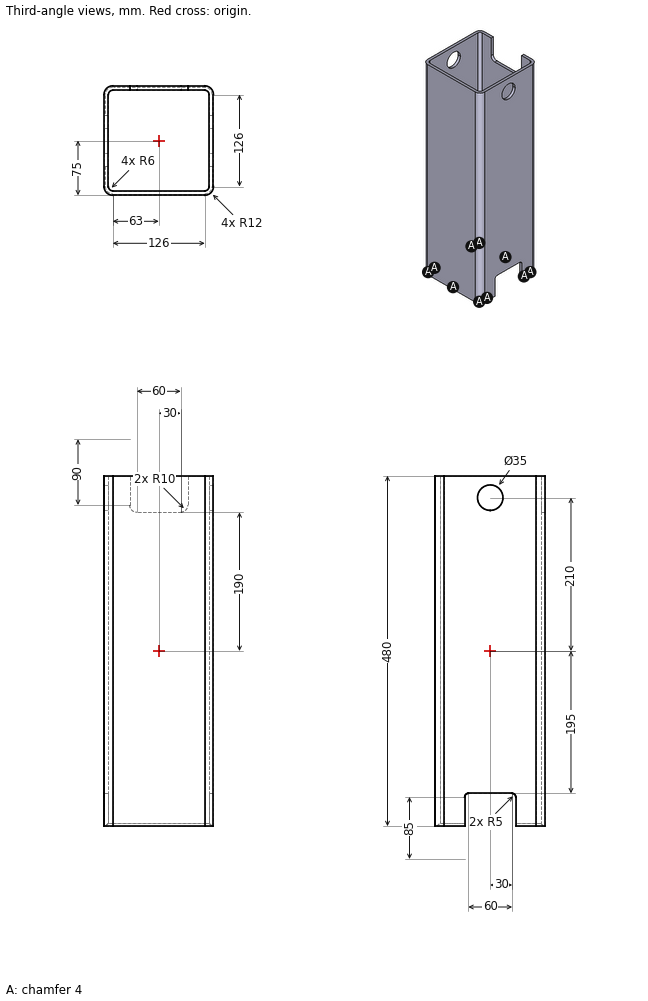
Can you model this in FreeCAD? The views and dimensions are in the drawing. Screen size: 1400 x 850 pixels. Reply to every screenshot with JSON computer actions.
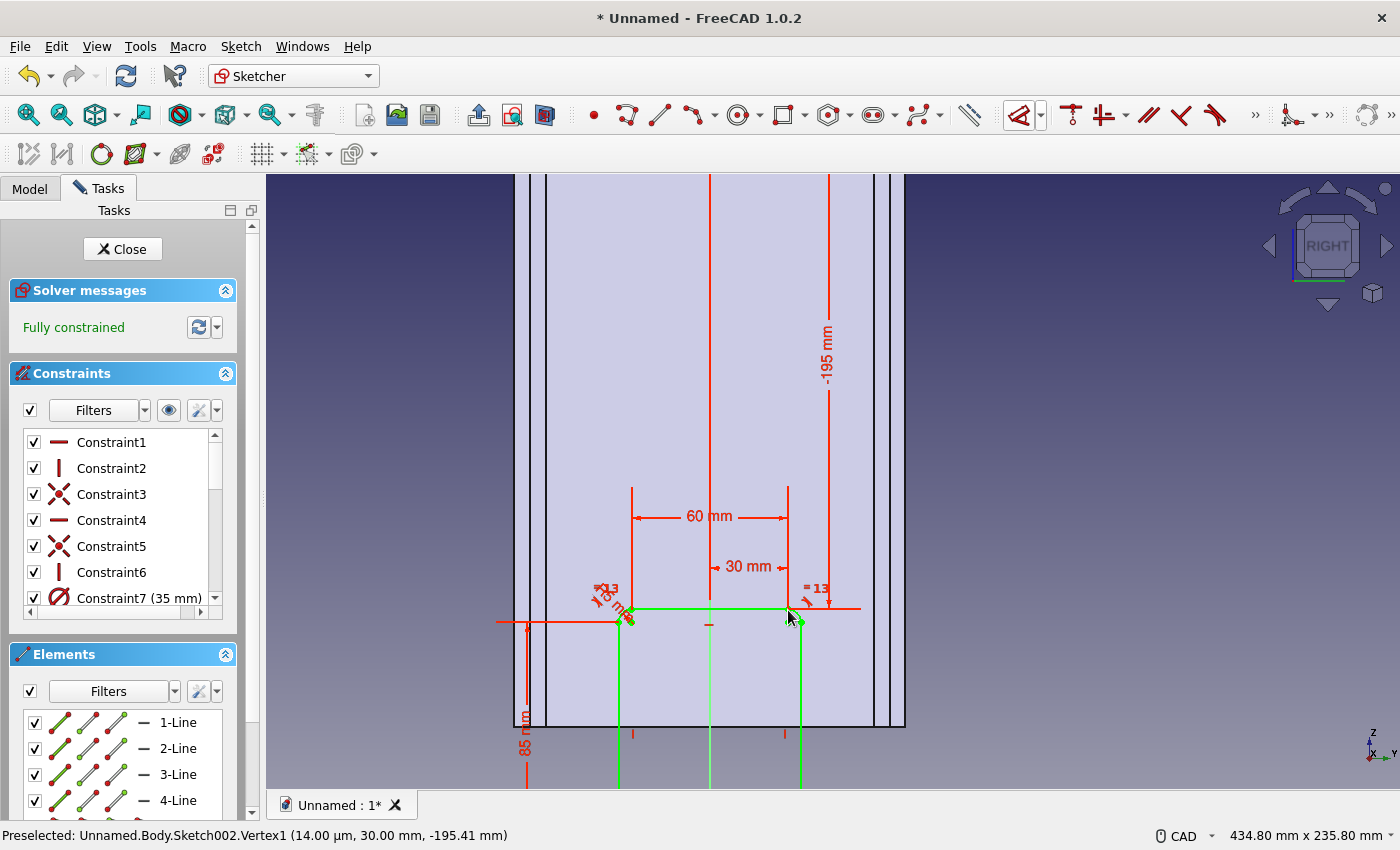
{"action": "left_click", "coordinate": [123, 249]}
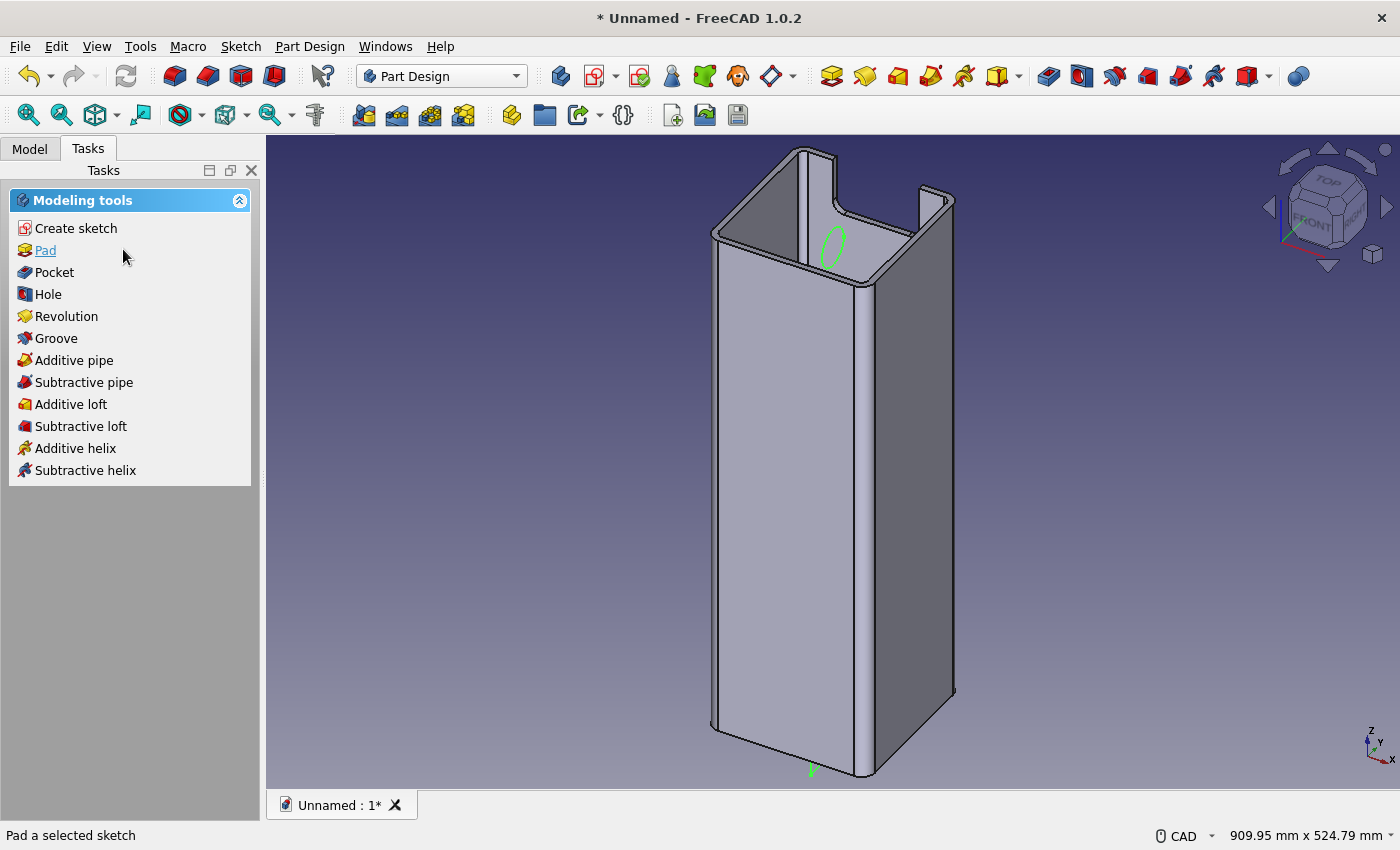
{"action": "left_click", "coordinate": [1049, 76]}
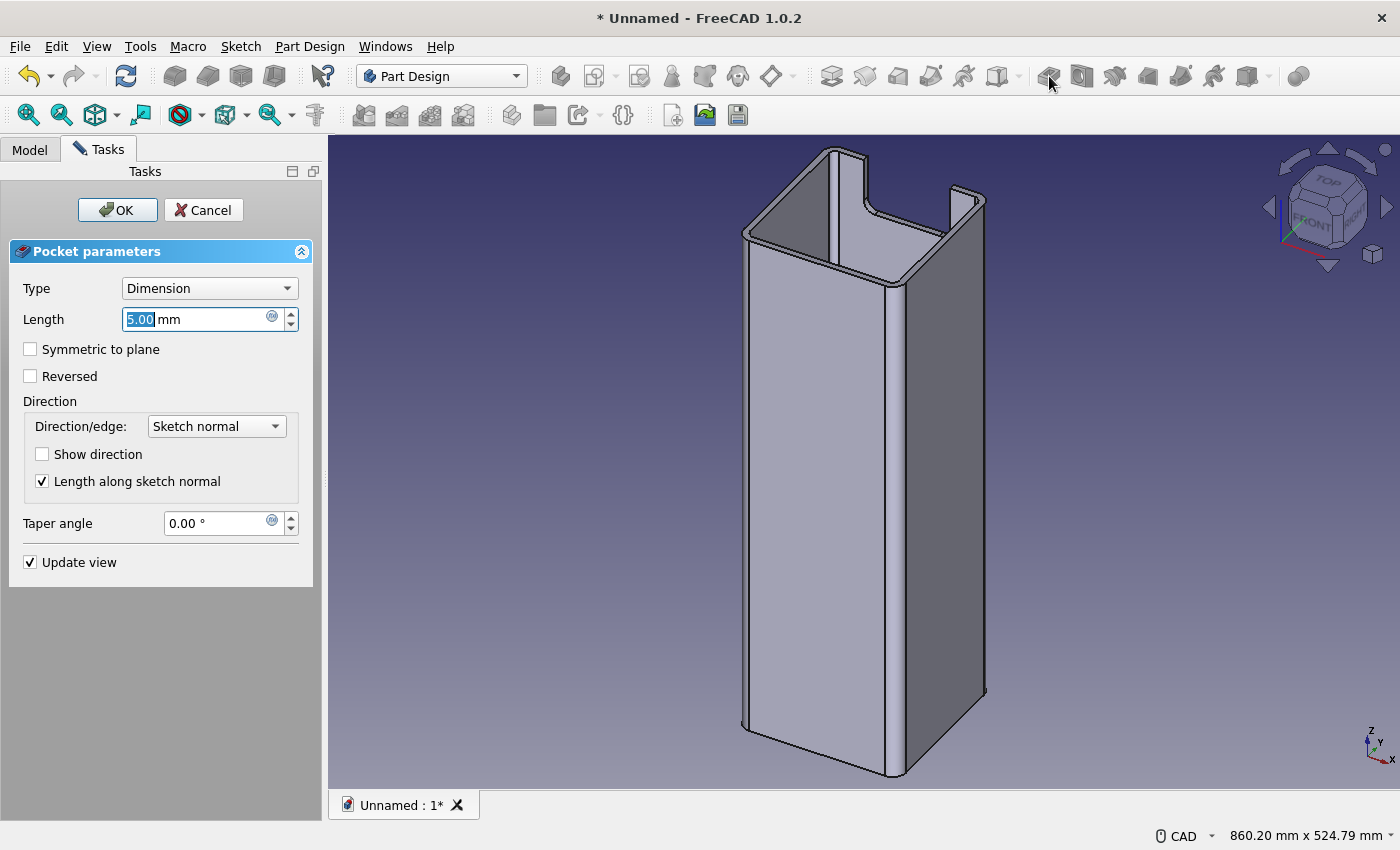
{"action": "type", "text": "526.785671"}
{"action": "key", "text": "Tab"}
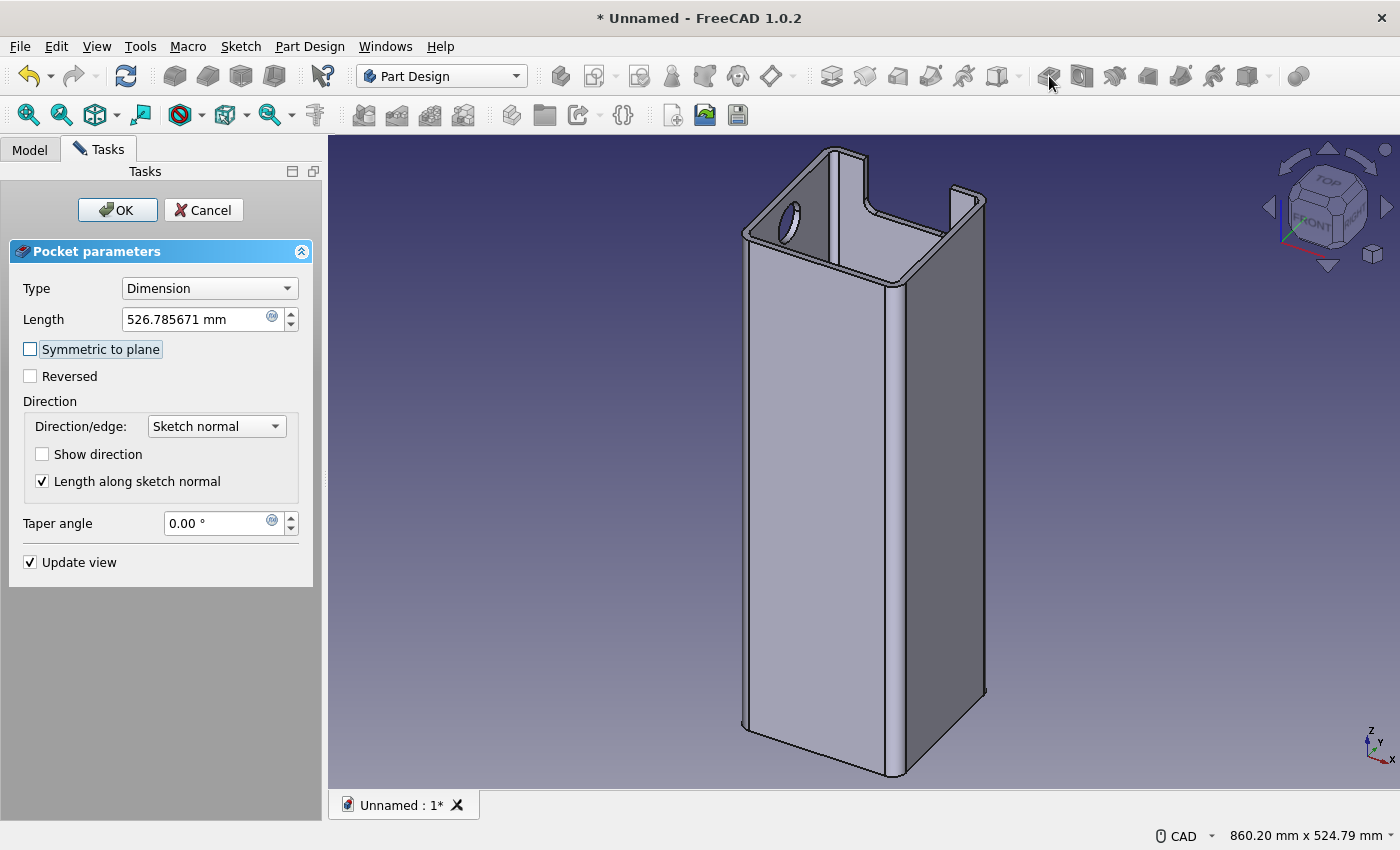
{"action": "left_click", "coordinate": [31, 349]}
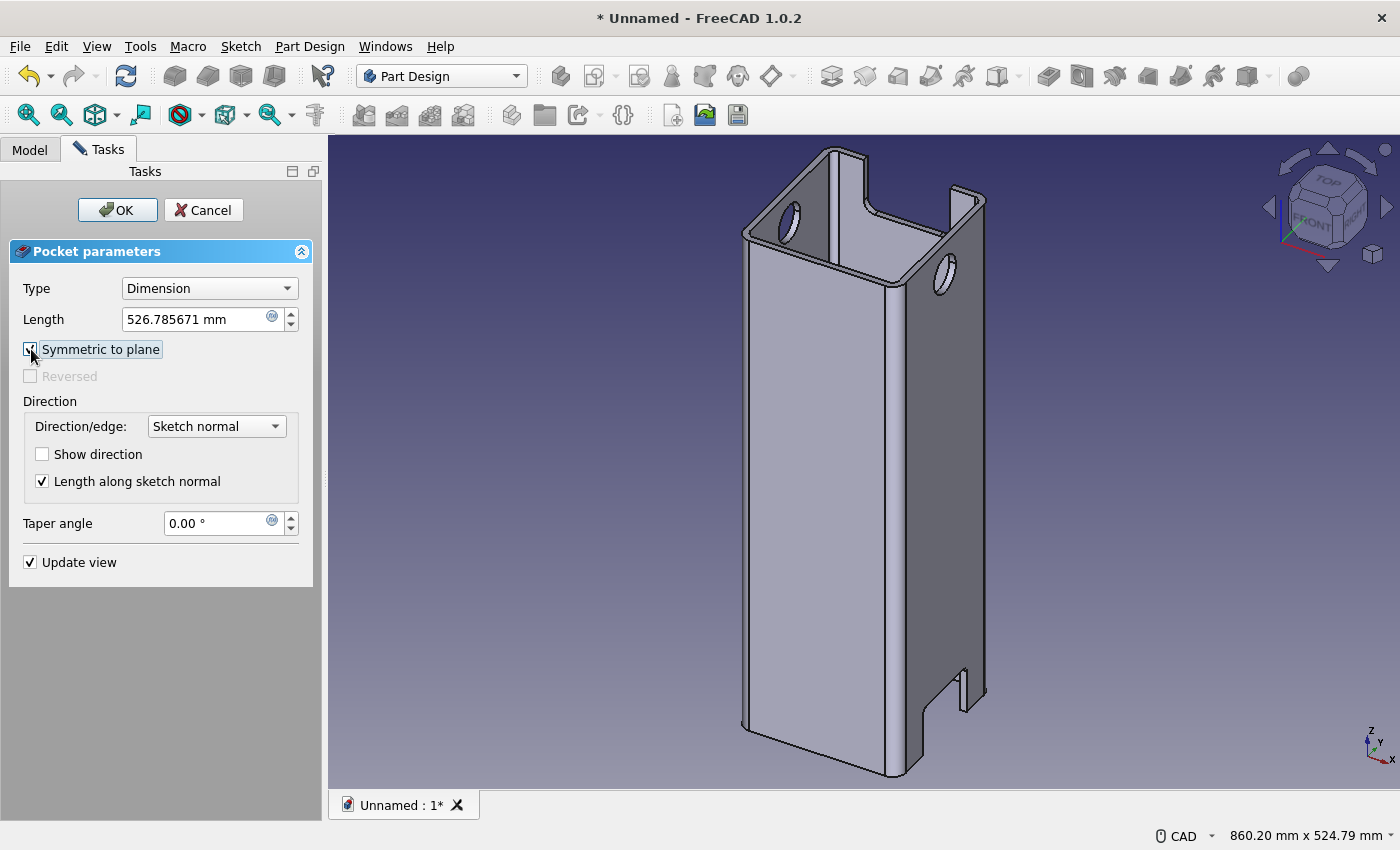
{"action": "left_click", "coordinate": [118, 210]}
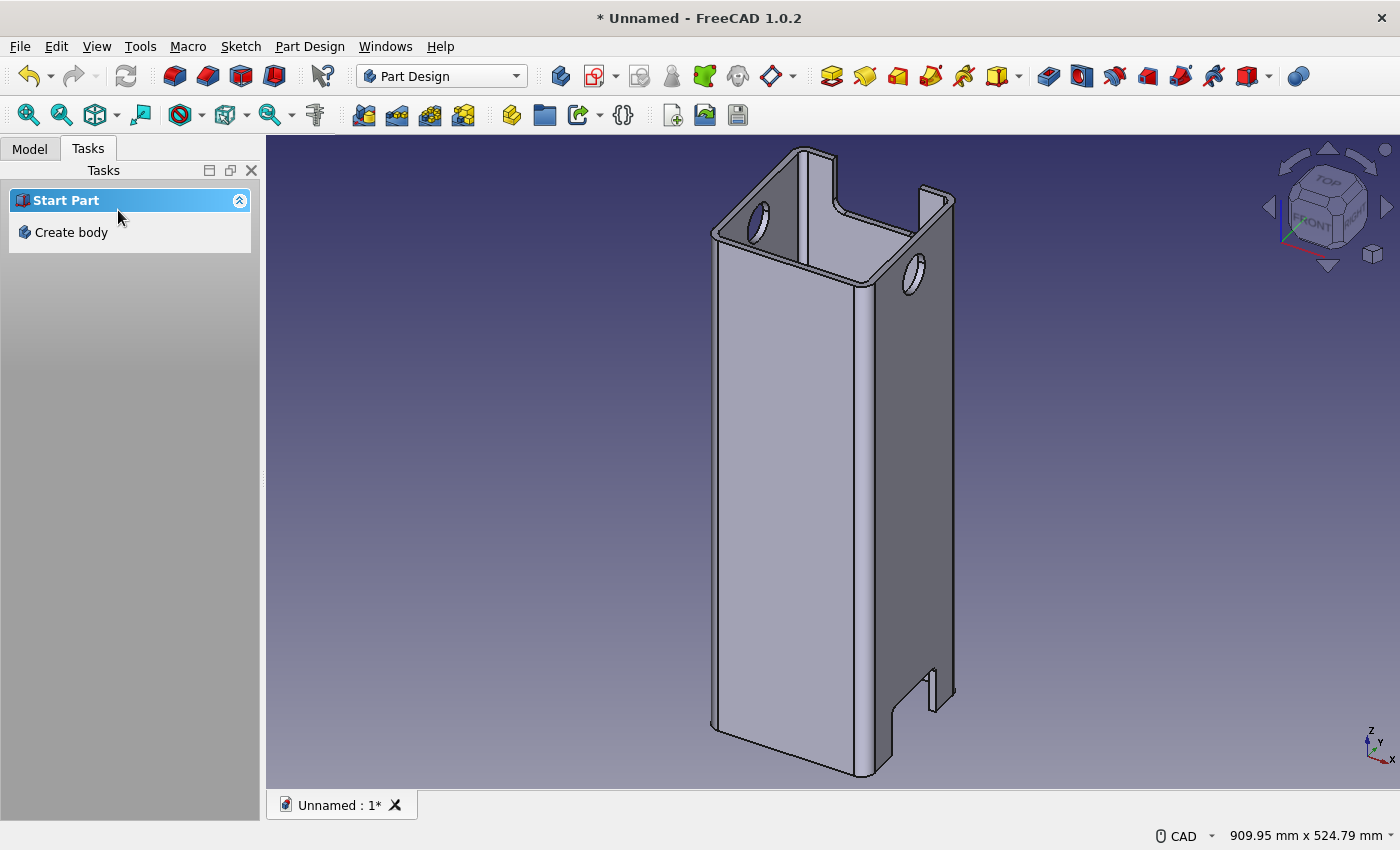
{"action": "scroll", "coordinate": [802, 640], "scroll_direction": "up", "scroll_amount": 7}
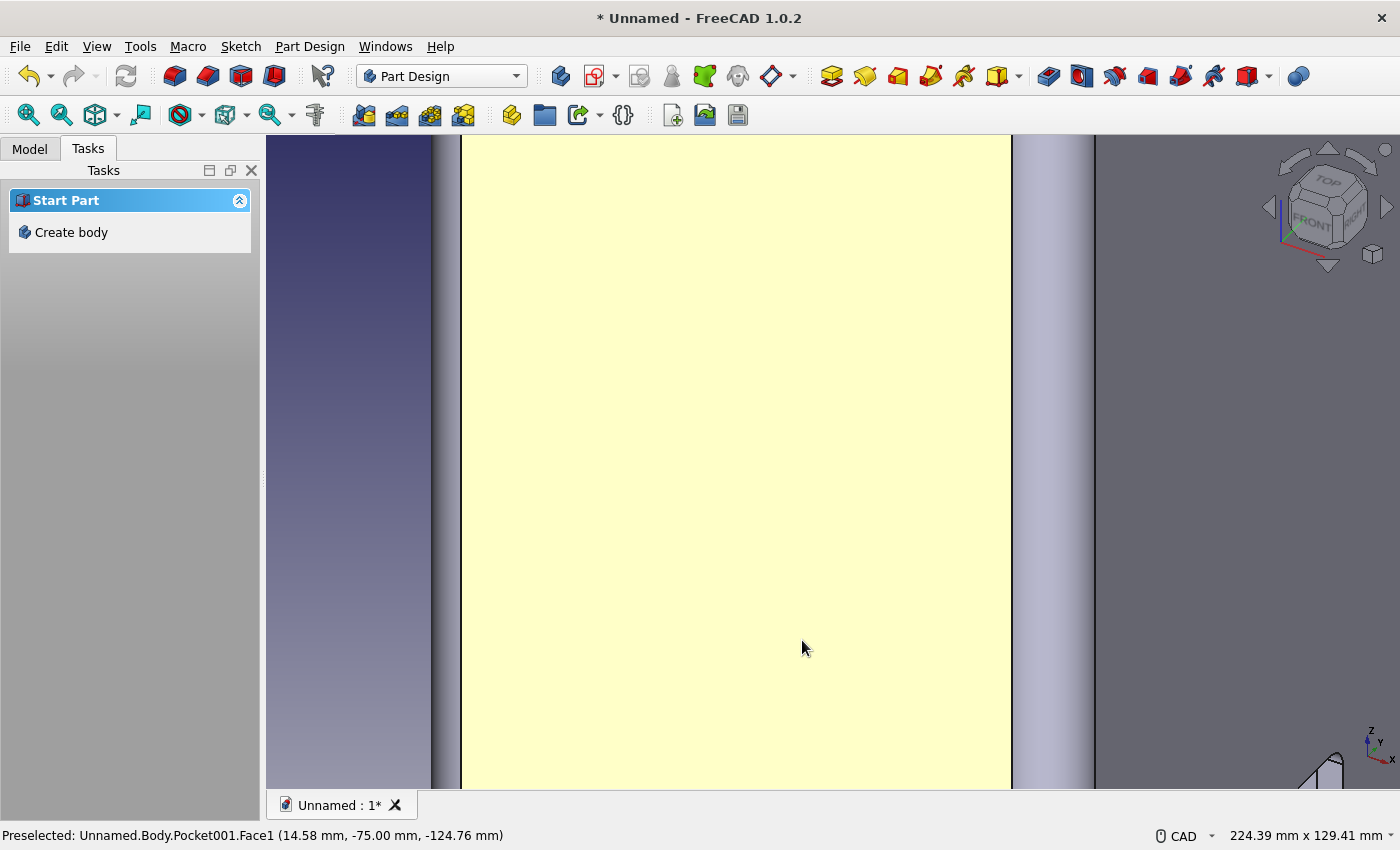
{"action": "left_click", "coordinate": [29, 116]}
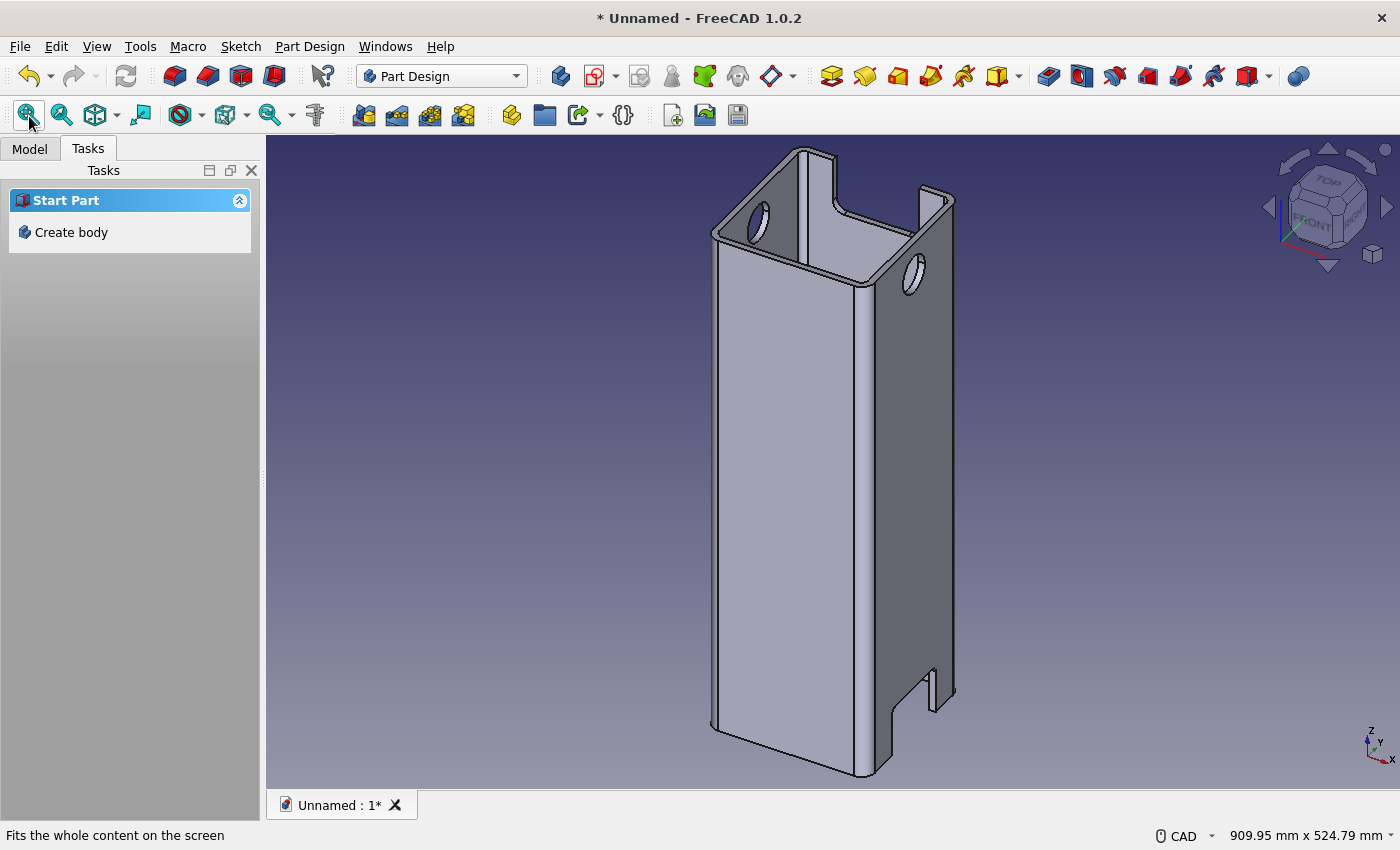
{"action": "key", "text": "0"}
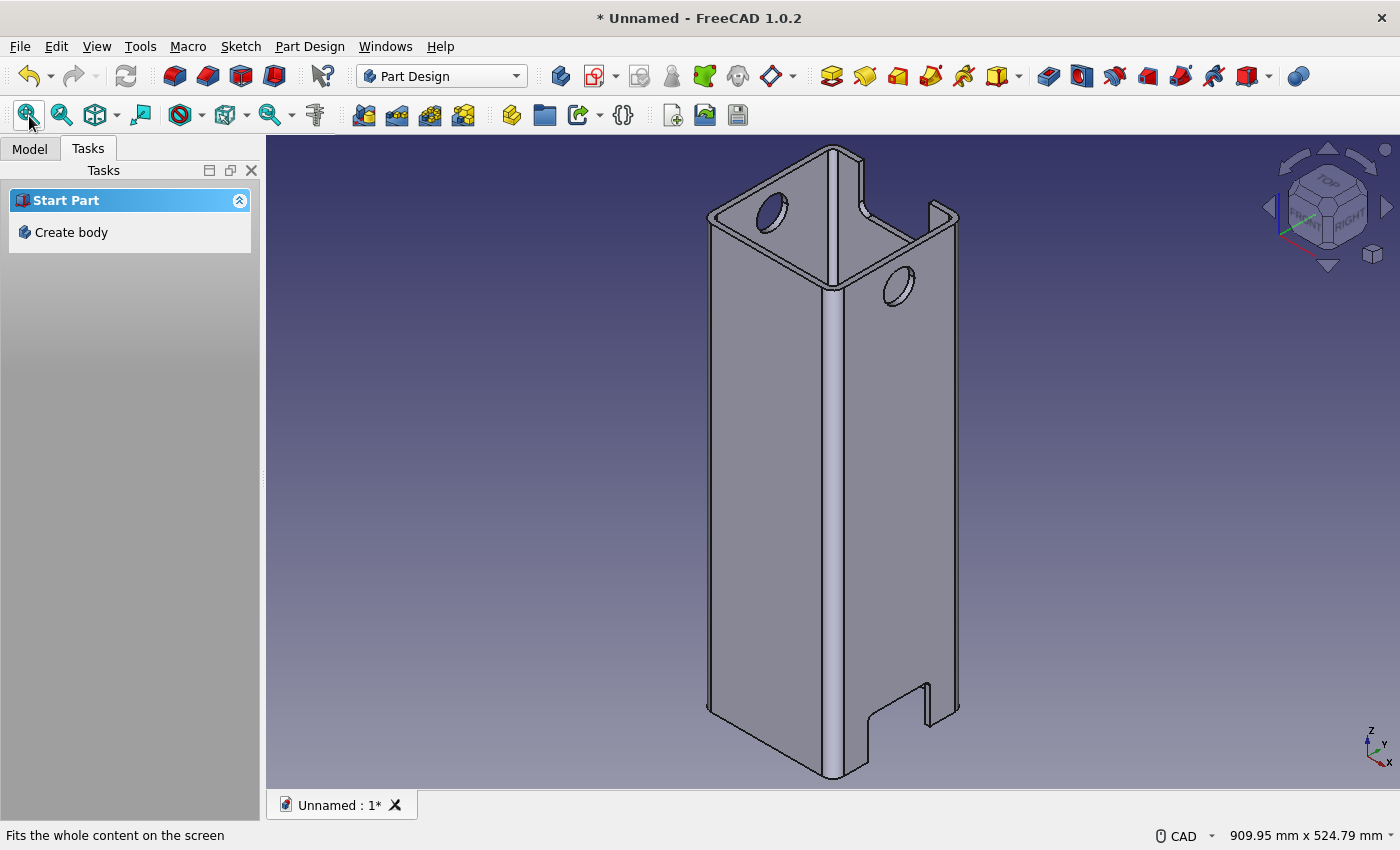
{"action": "scroll", "coordinate": [833, 637], "scroll_direction": "up", "scroll_amount": 7}